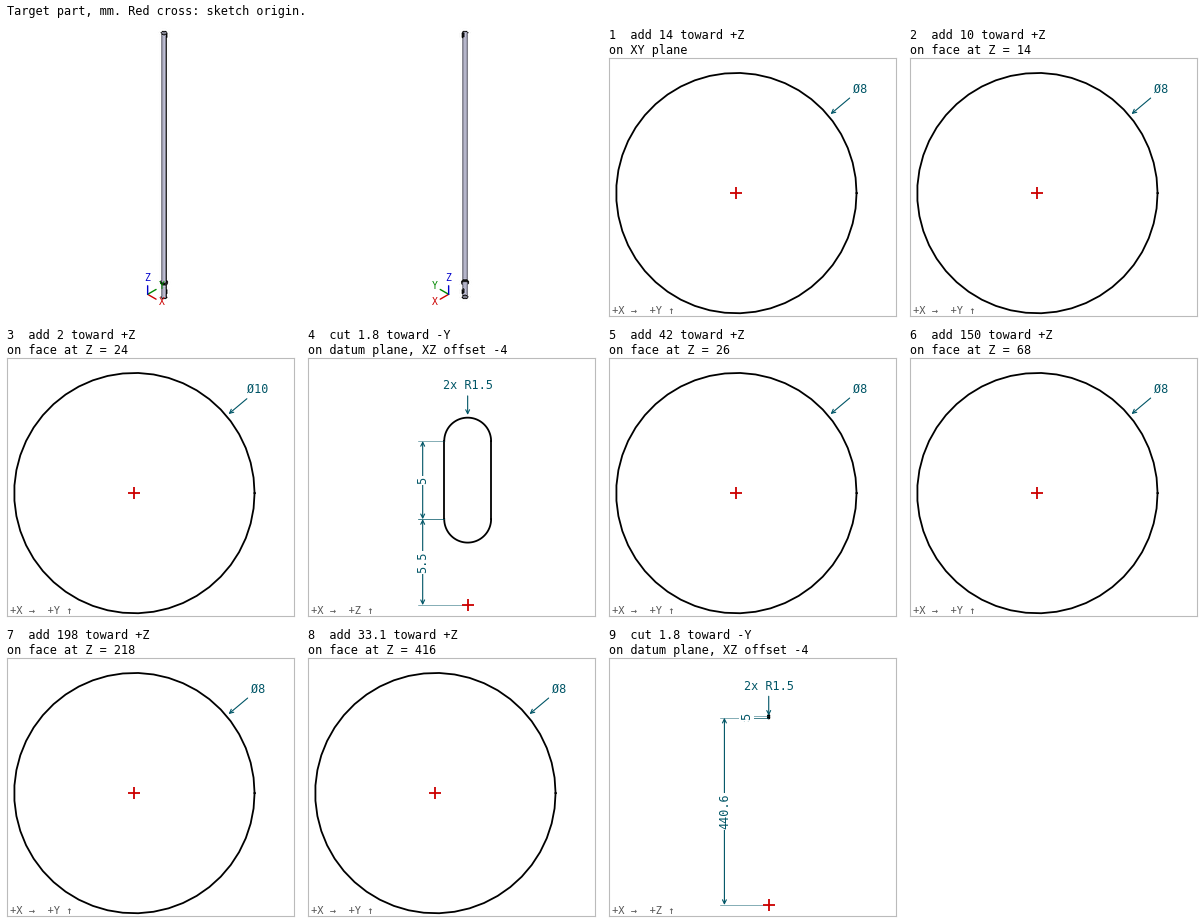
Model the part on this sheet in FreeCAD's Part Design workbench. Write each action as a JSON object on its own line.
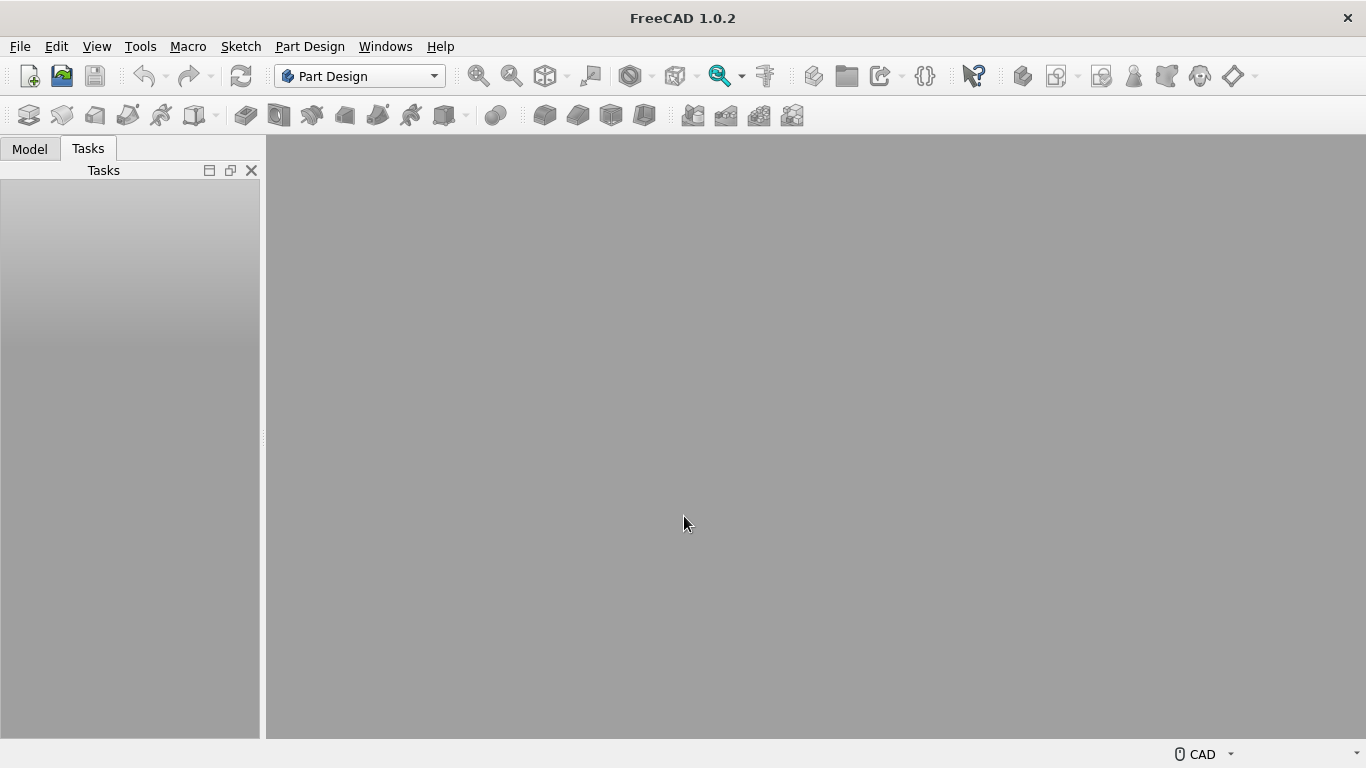
{"action": "left_click", "coordinate": [29, 76]}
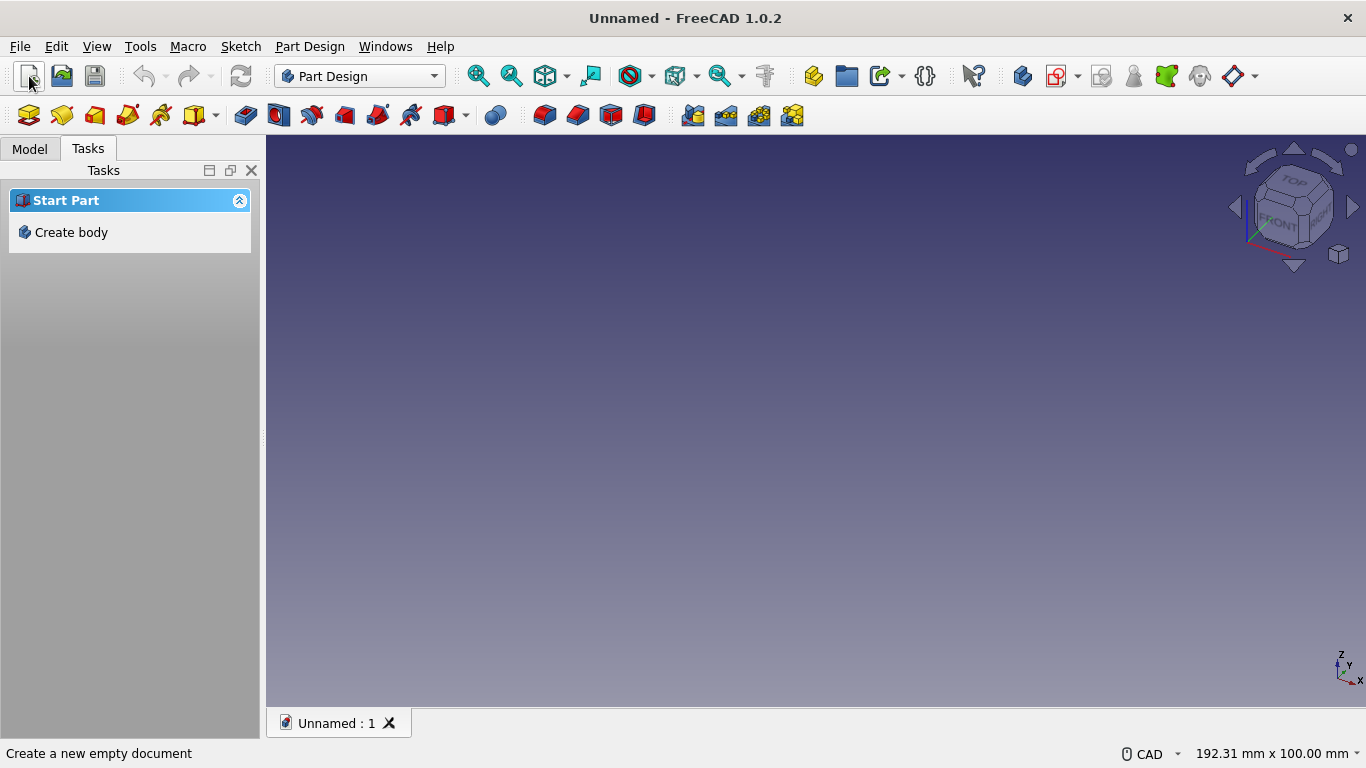
{"action": "left_click", "coordinate": [1056, 76]}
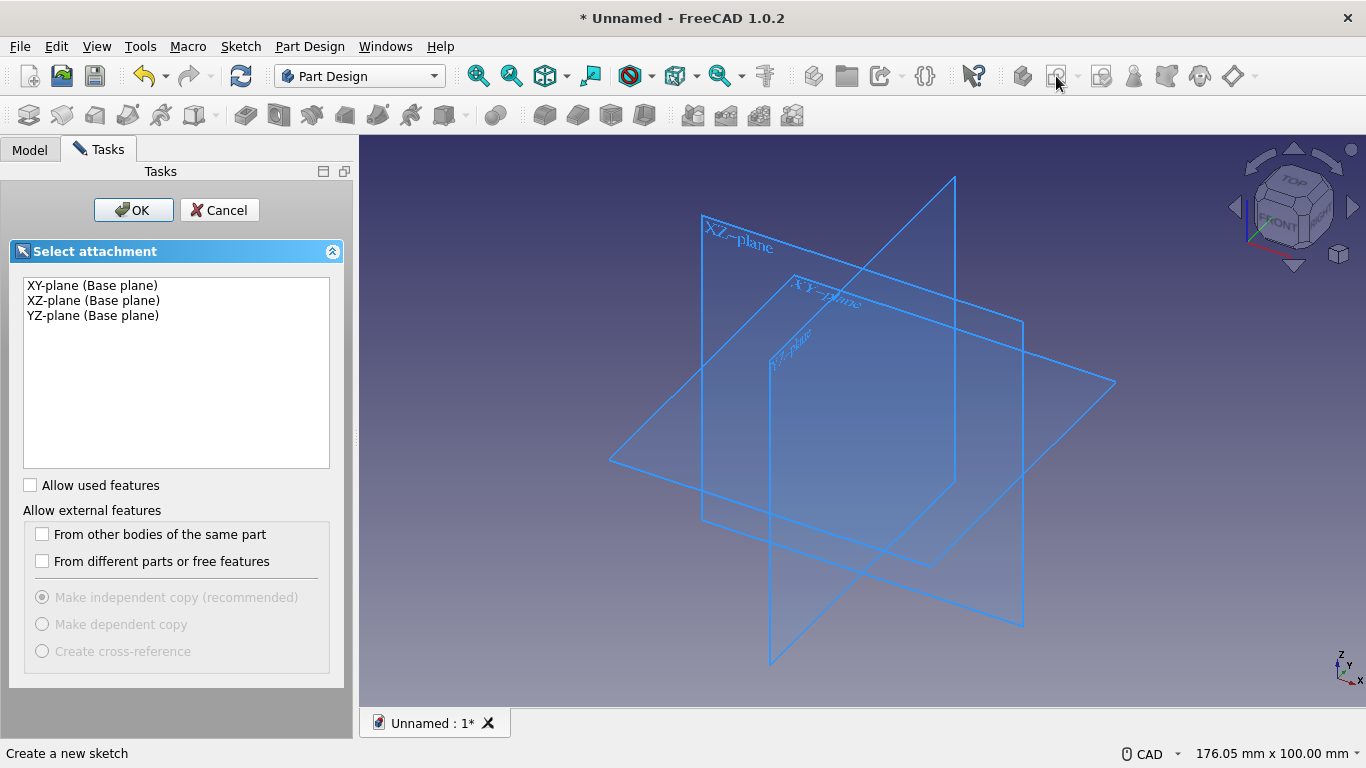
{"action": "left_click", "coordinate": [84, 286]}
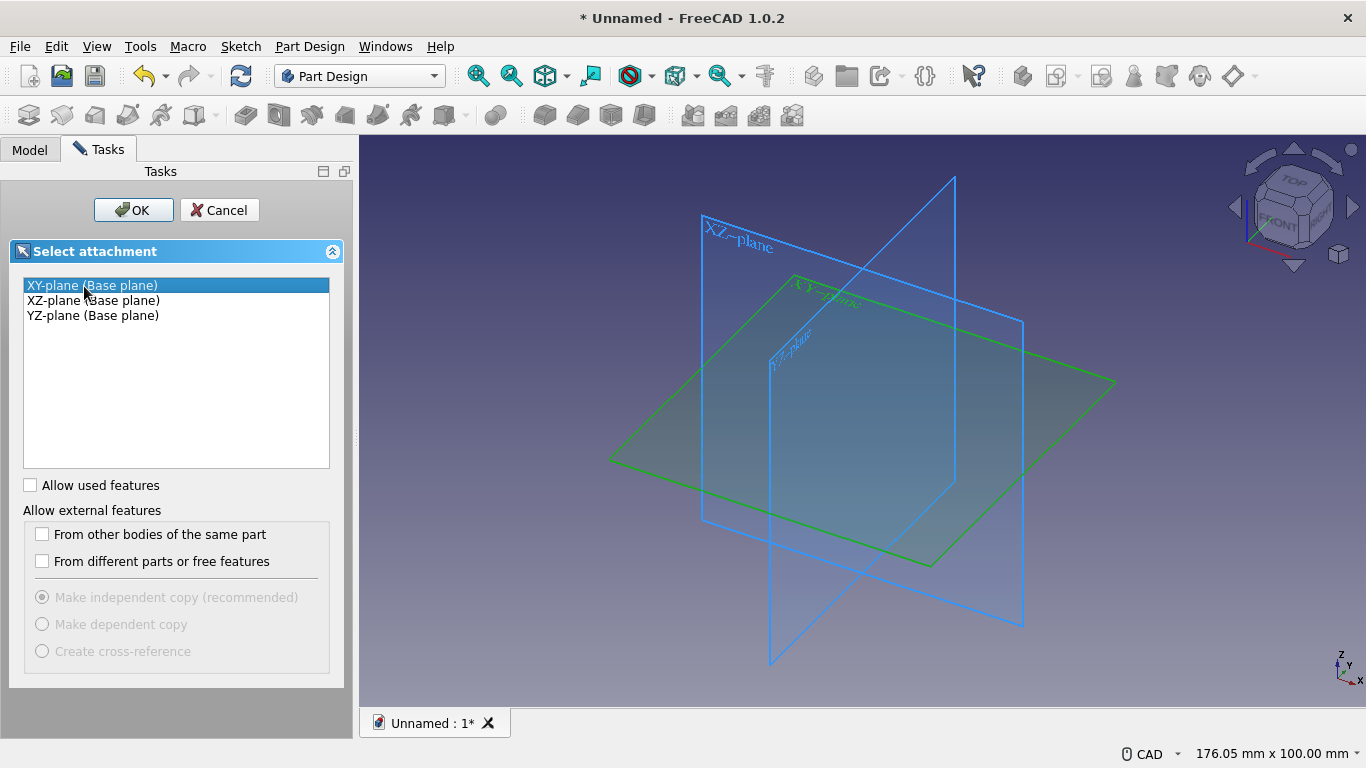
{"action": "left_click", "coordinate": [134, 210]}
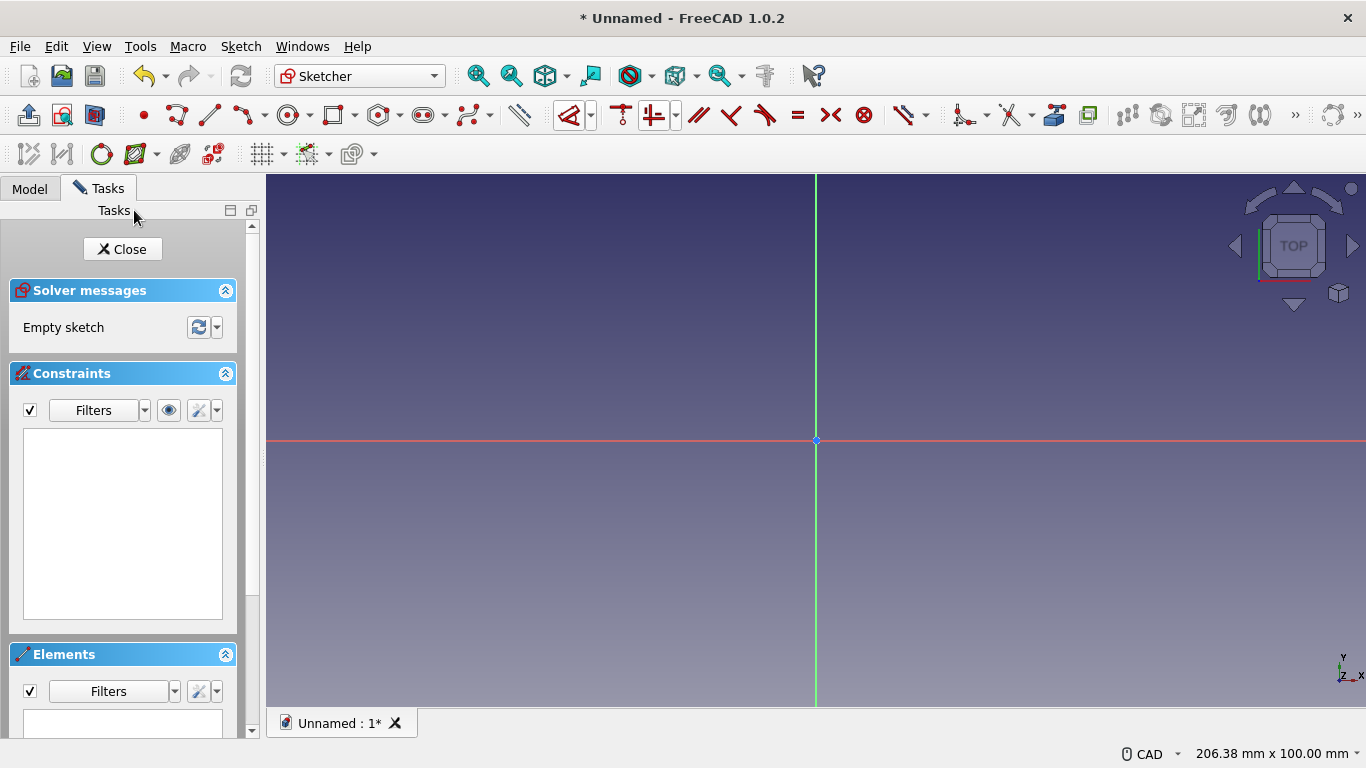
{"action": "scroll", "coordinate": [827, 440], "scroll_direction": "up", "scroll_amount": 10}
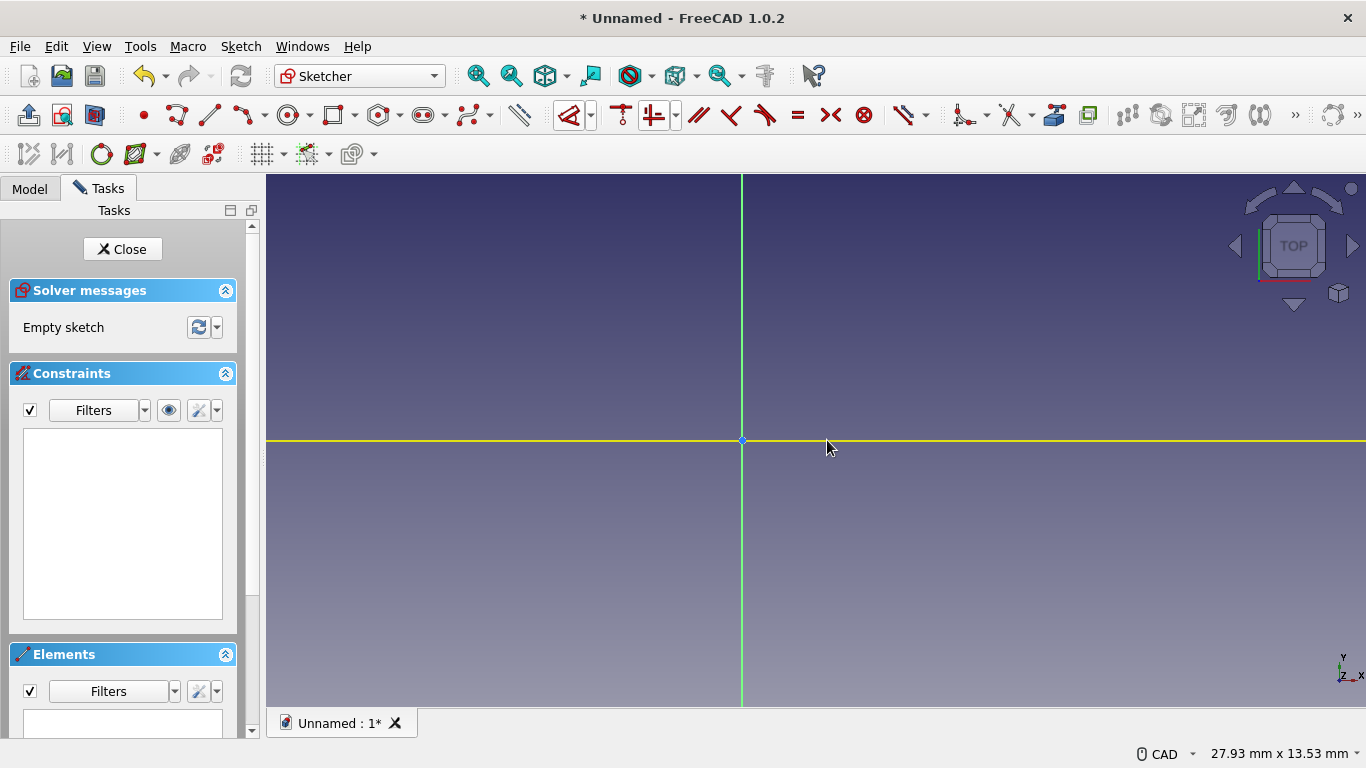
{"action": "left_click", "coordinate": [288, 116]}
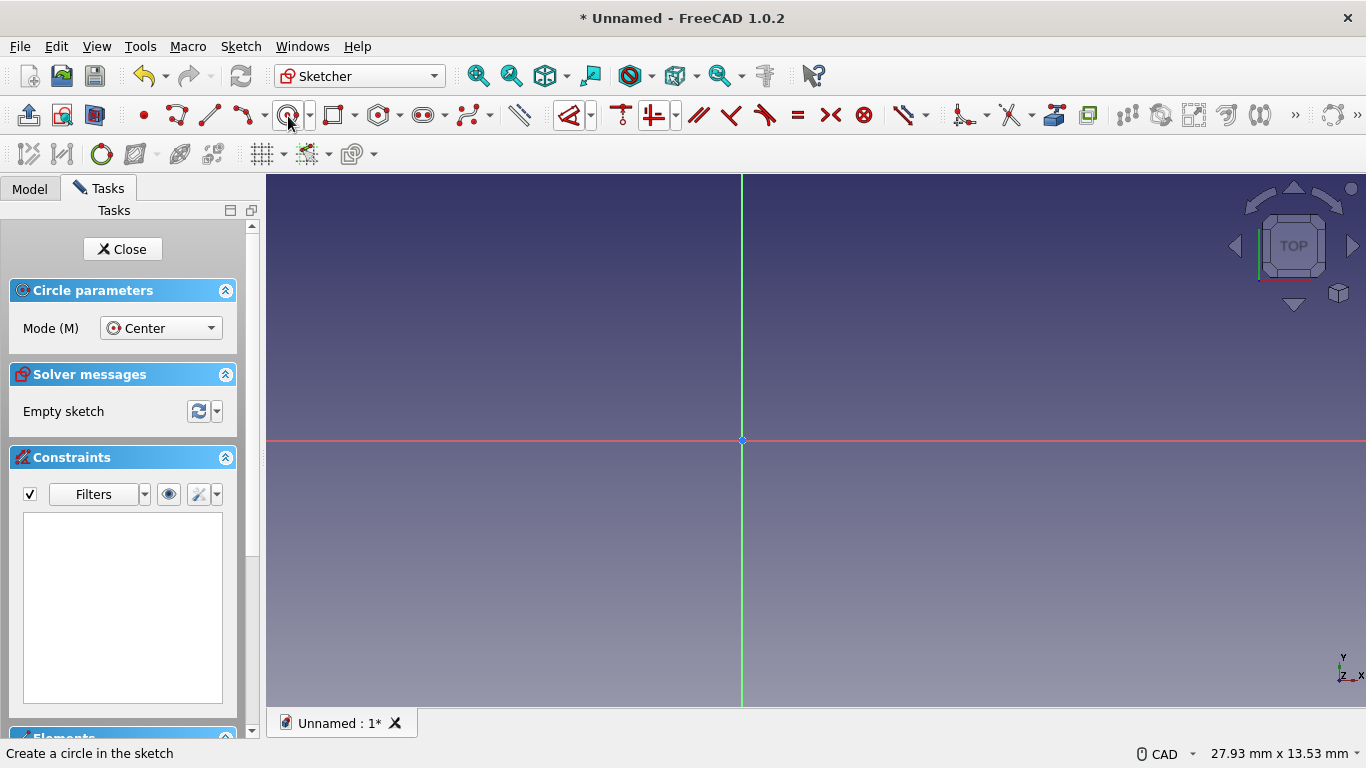
{"action": "left_click", "coordinate": [742, 440]}
{"action": "left_click", "coordinate": [854, 329]}
{"action": "key", "text": "Escape"}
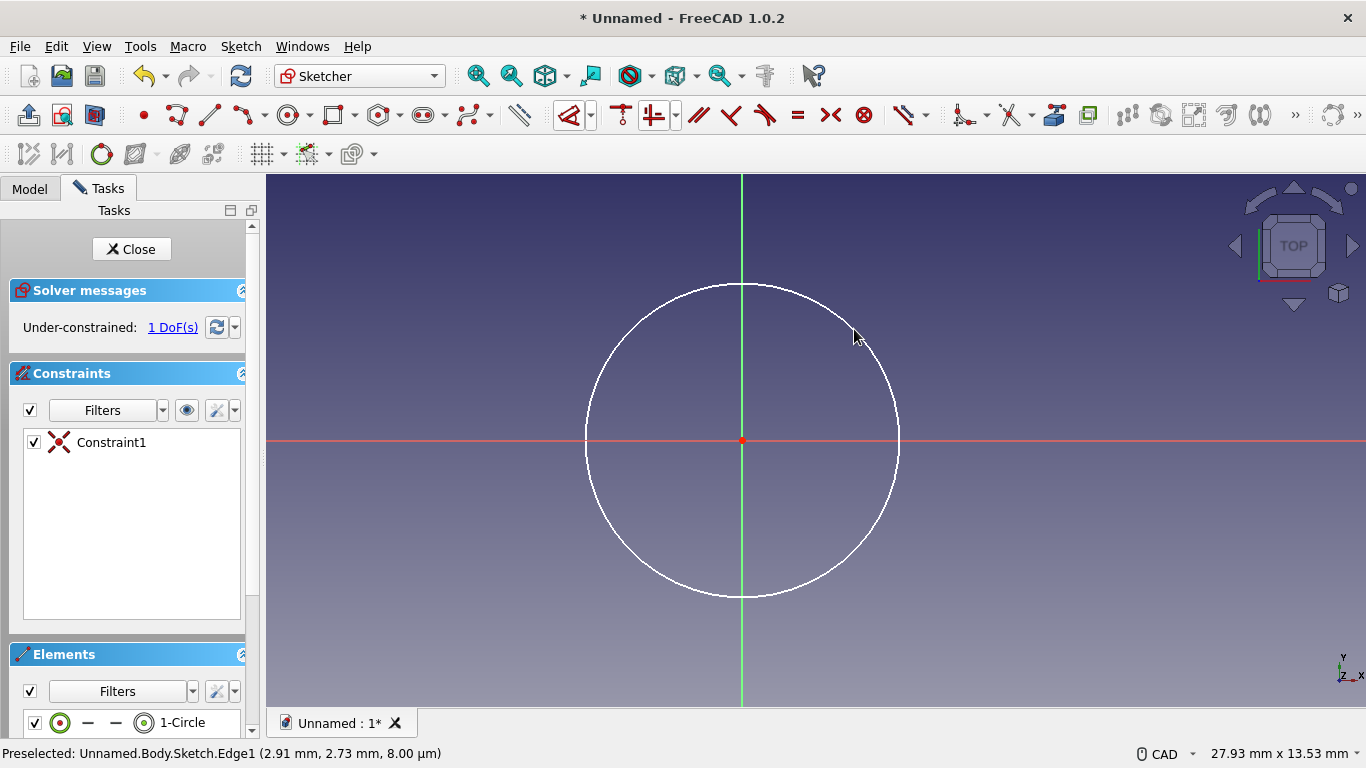
{"action": "left_click", "coordinate": [853, 329]}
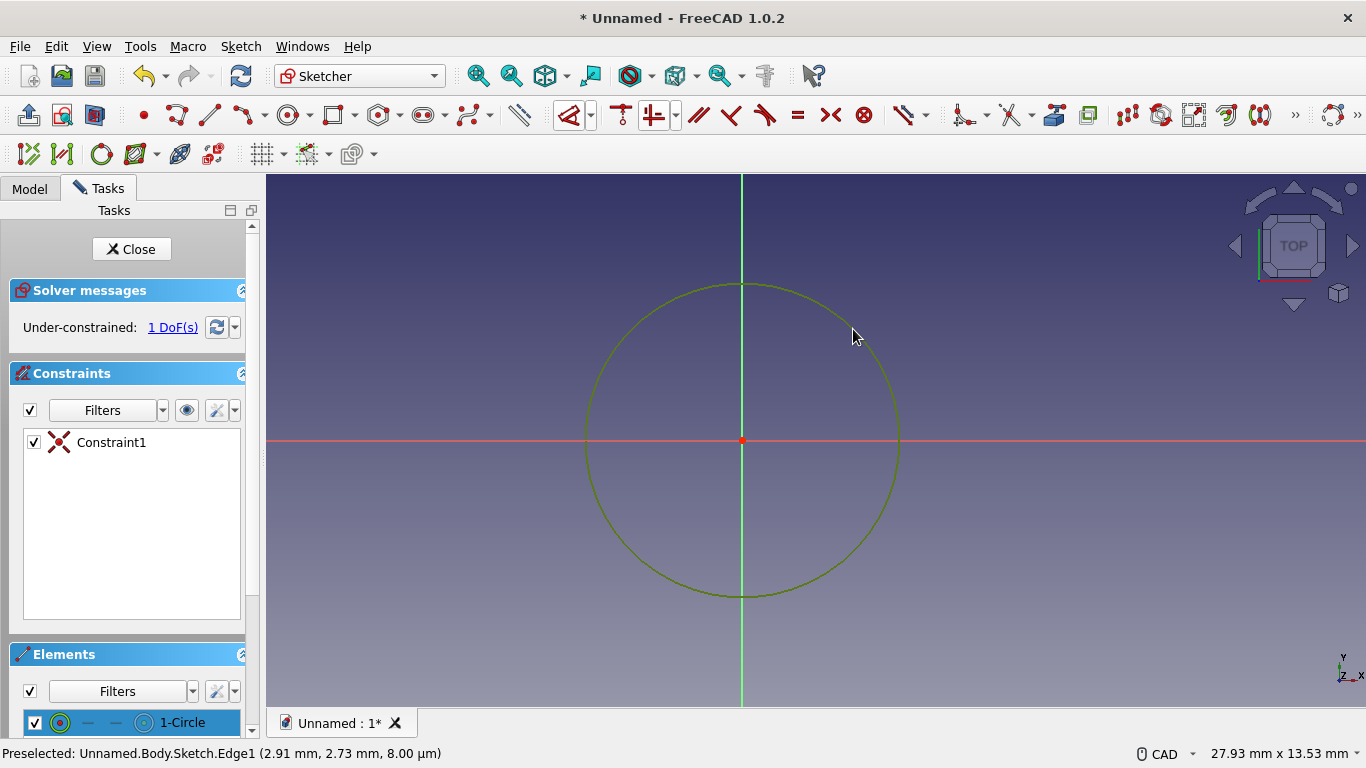
{"action": "left_click", "coordinate": [590, 116]}